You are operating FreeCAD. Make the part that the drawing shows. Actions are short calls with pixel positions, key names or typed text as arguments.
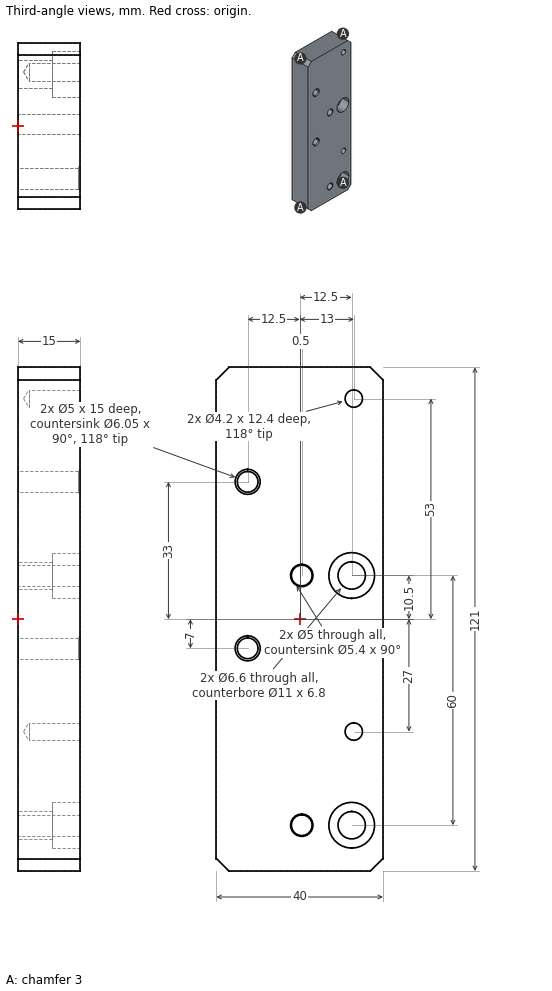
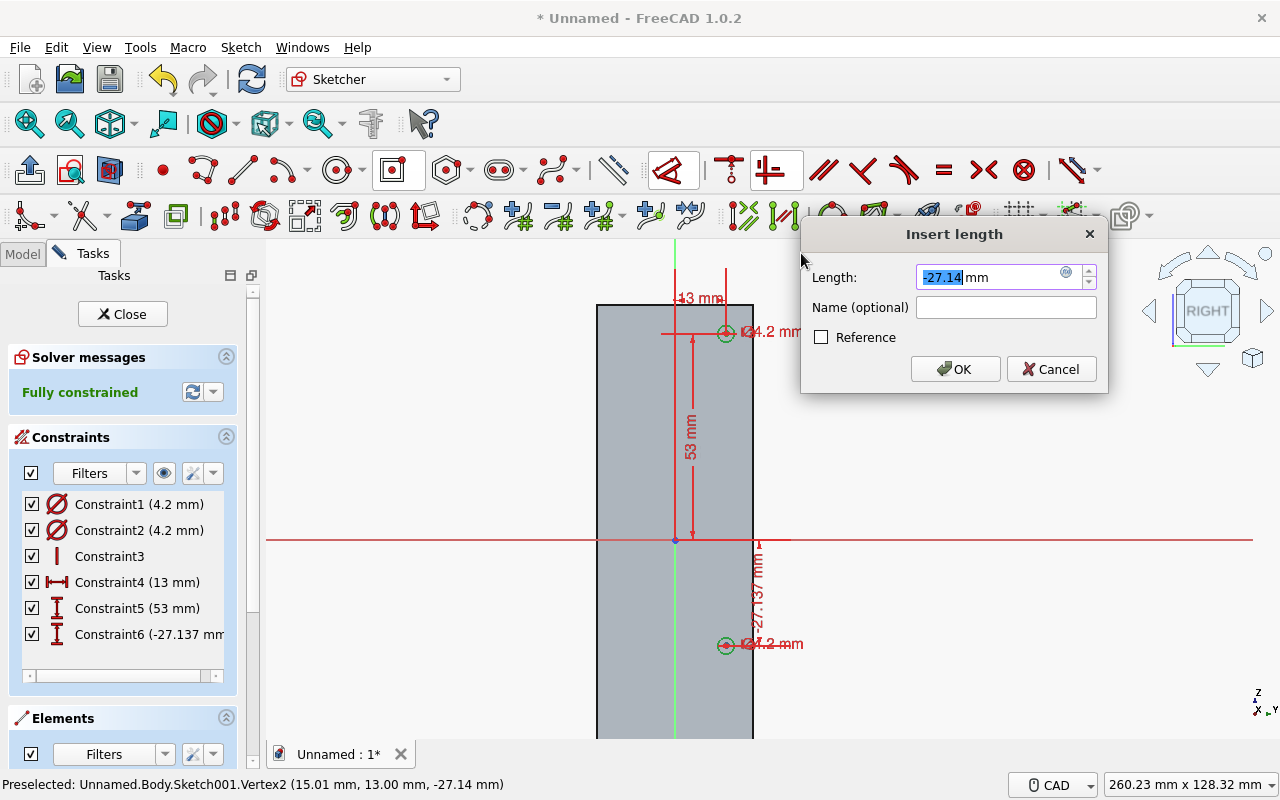
text(-27)
key(Return)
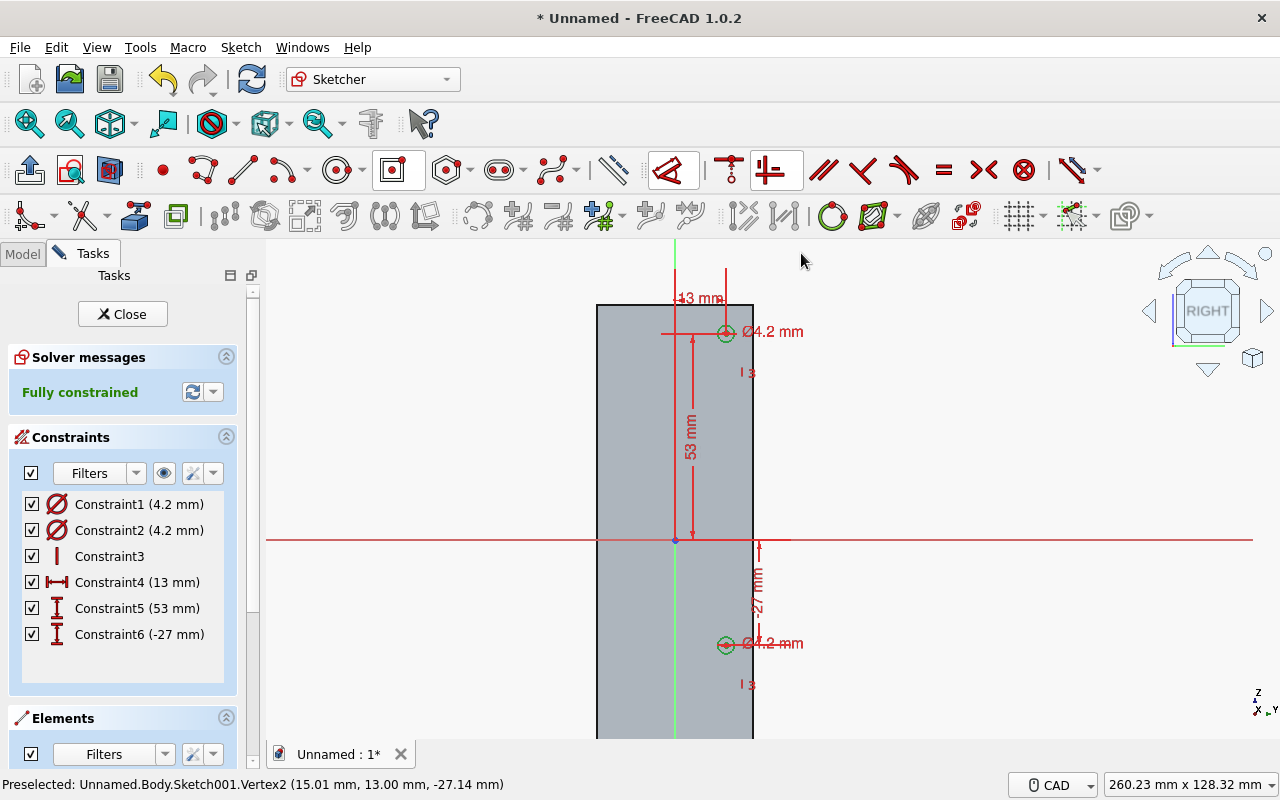
click(123, 314)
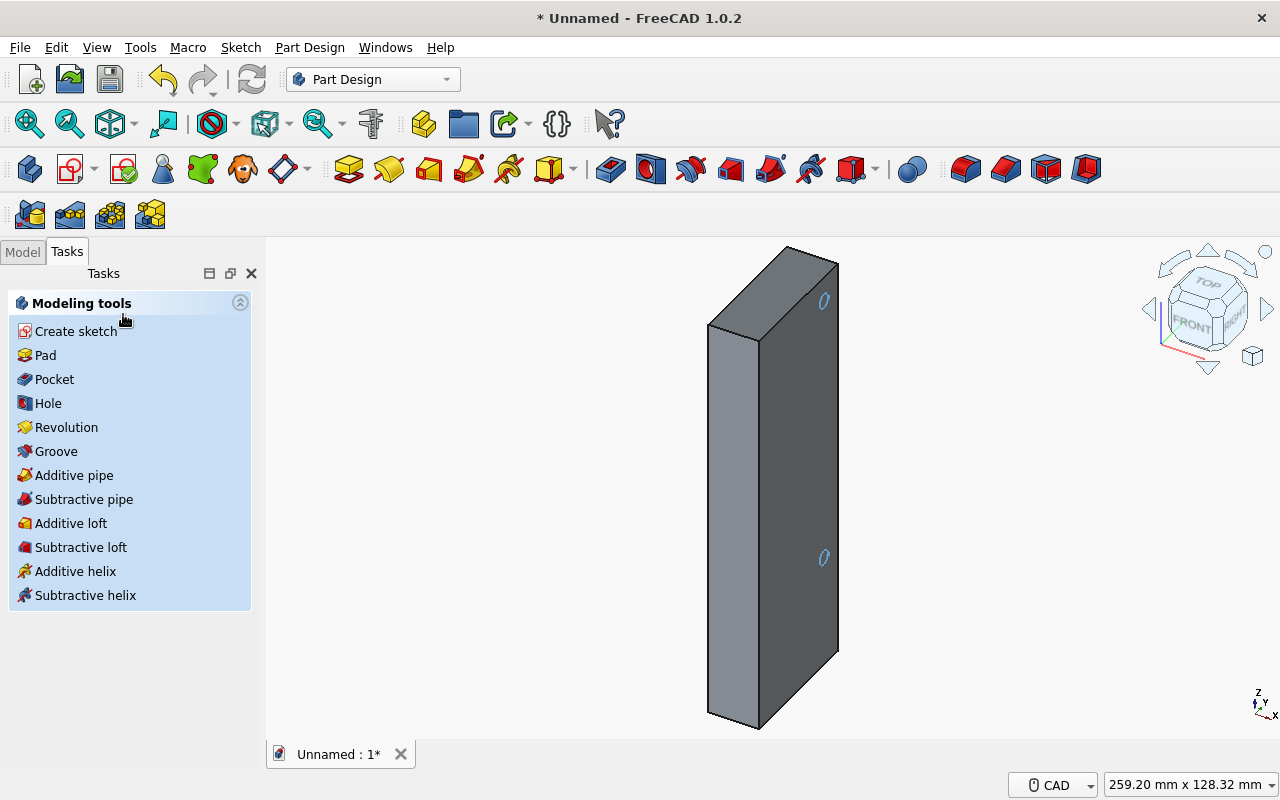
click(652, 170)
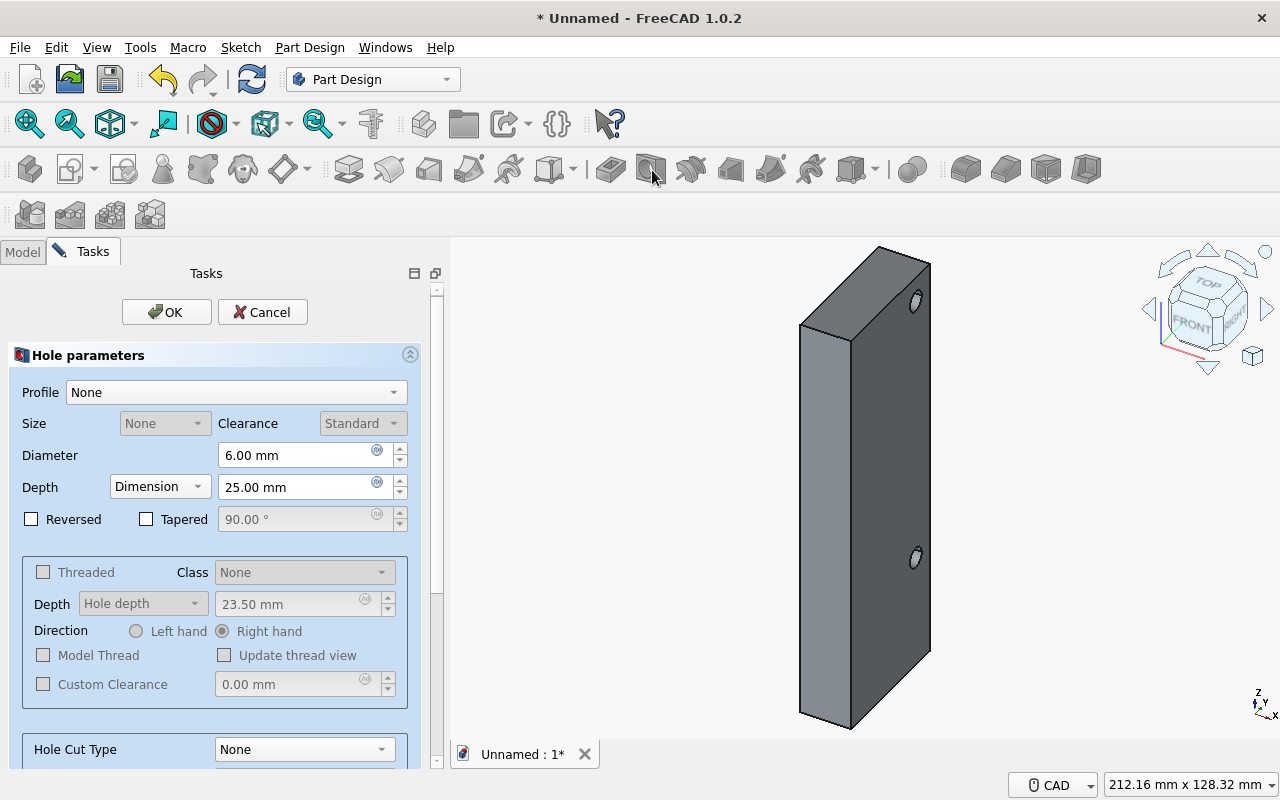
triple_click(305, 455)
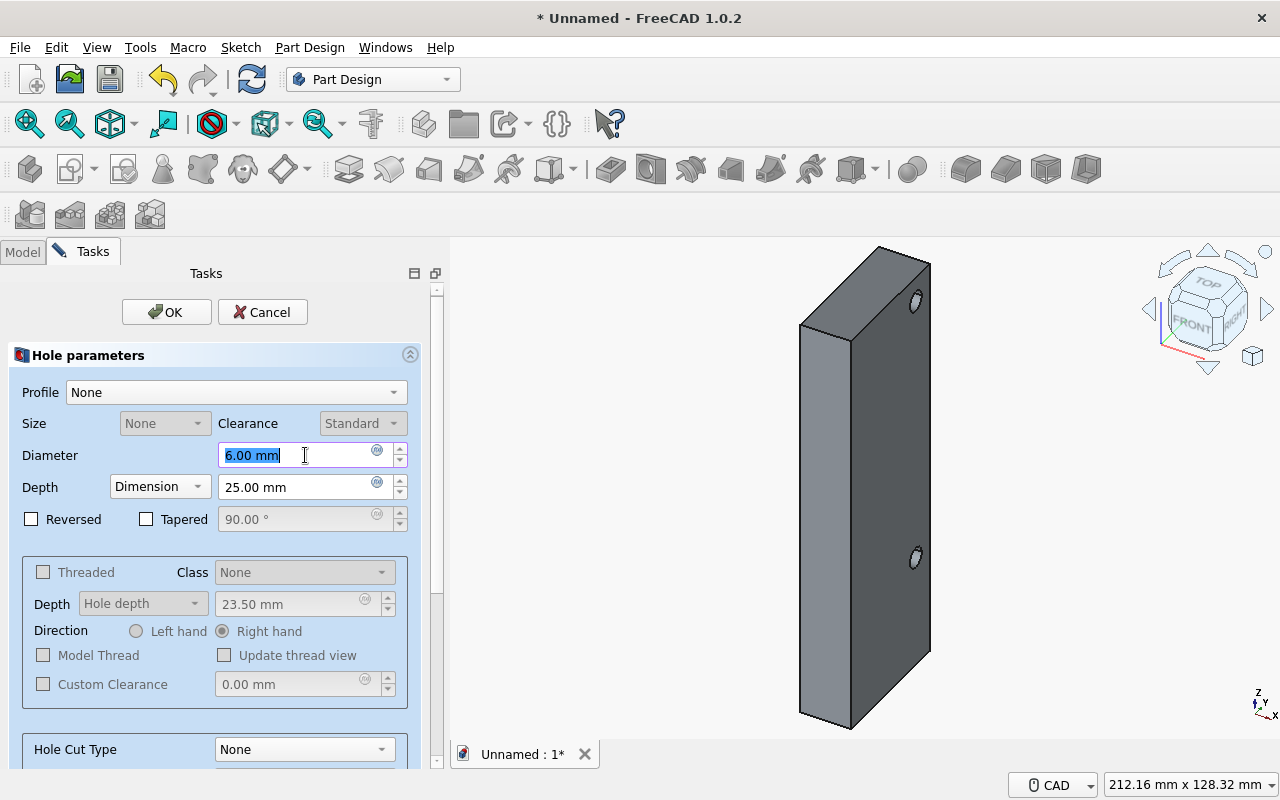
text(4.2)
key(Tab)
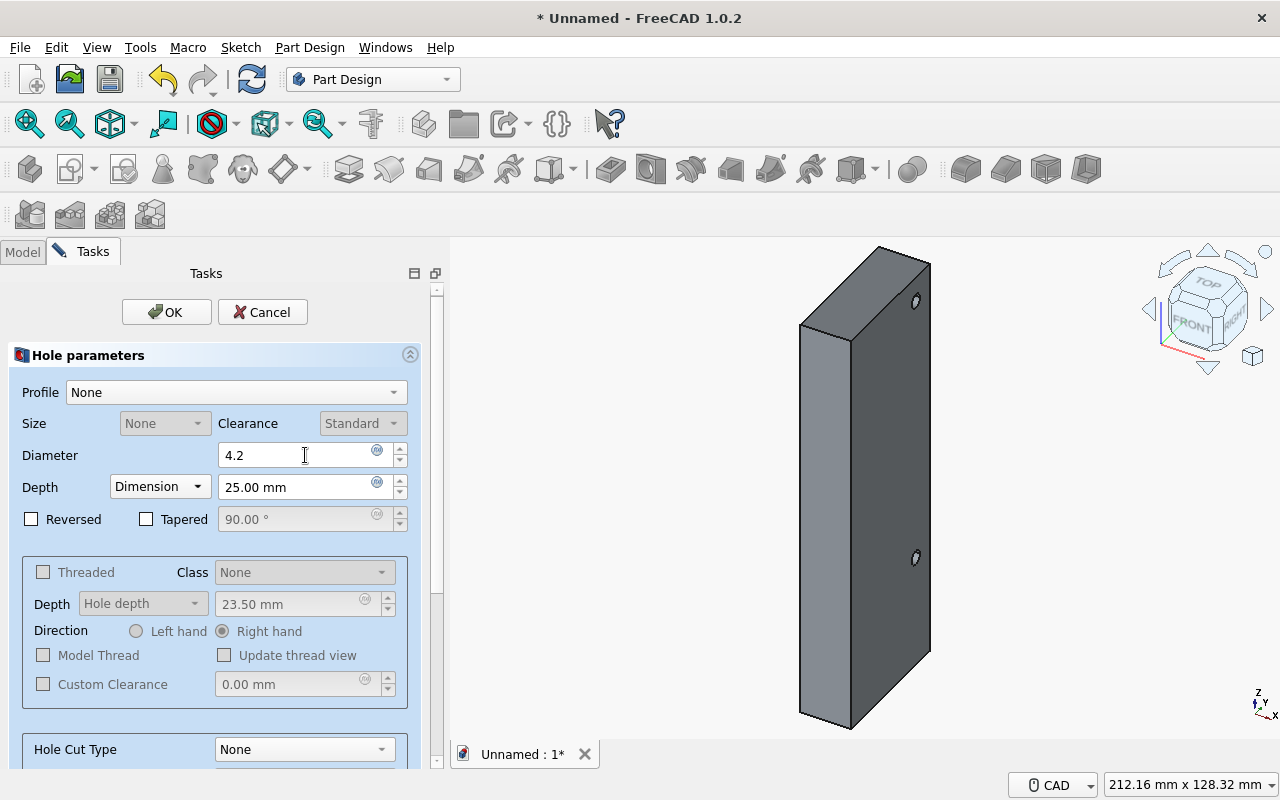
triple_click(305, 487)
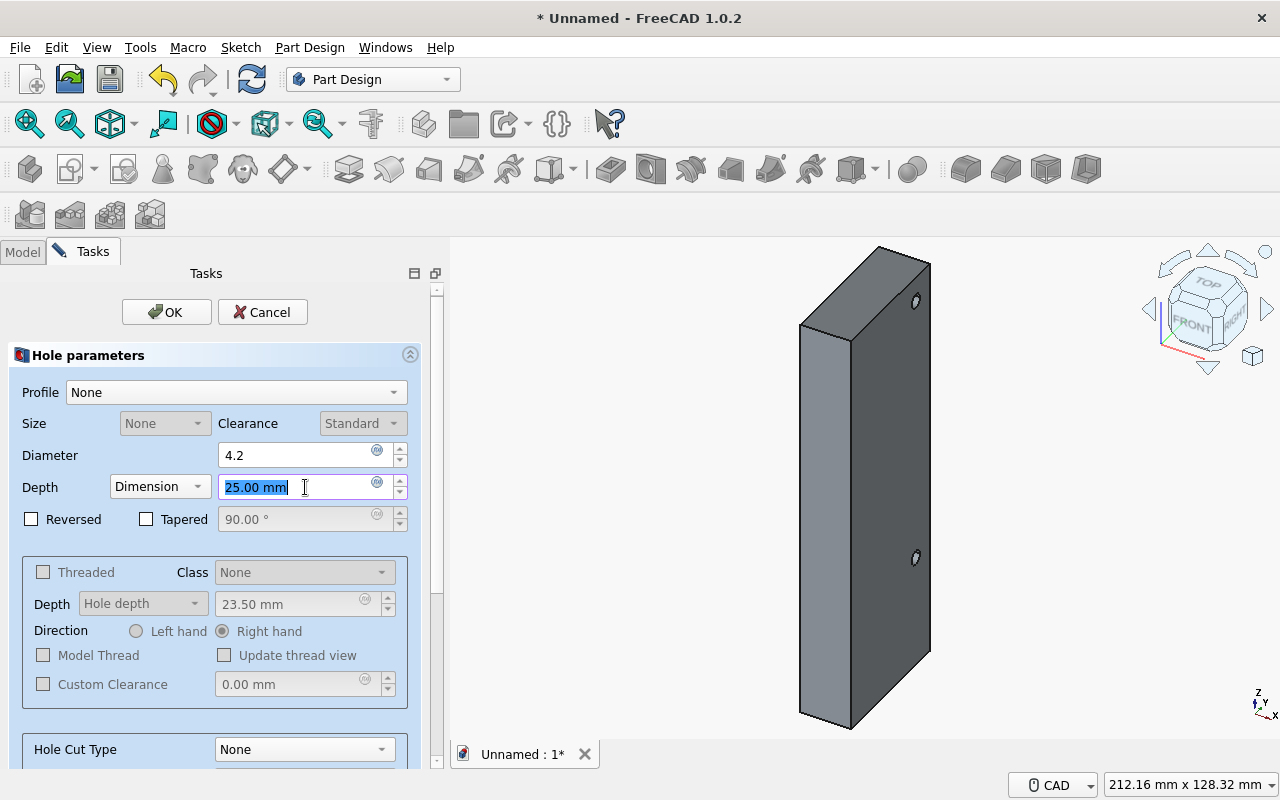
text(12.4)
key(Tab)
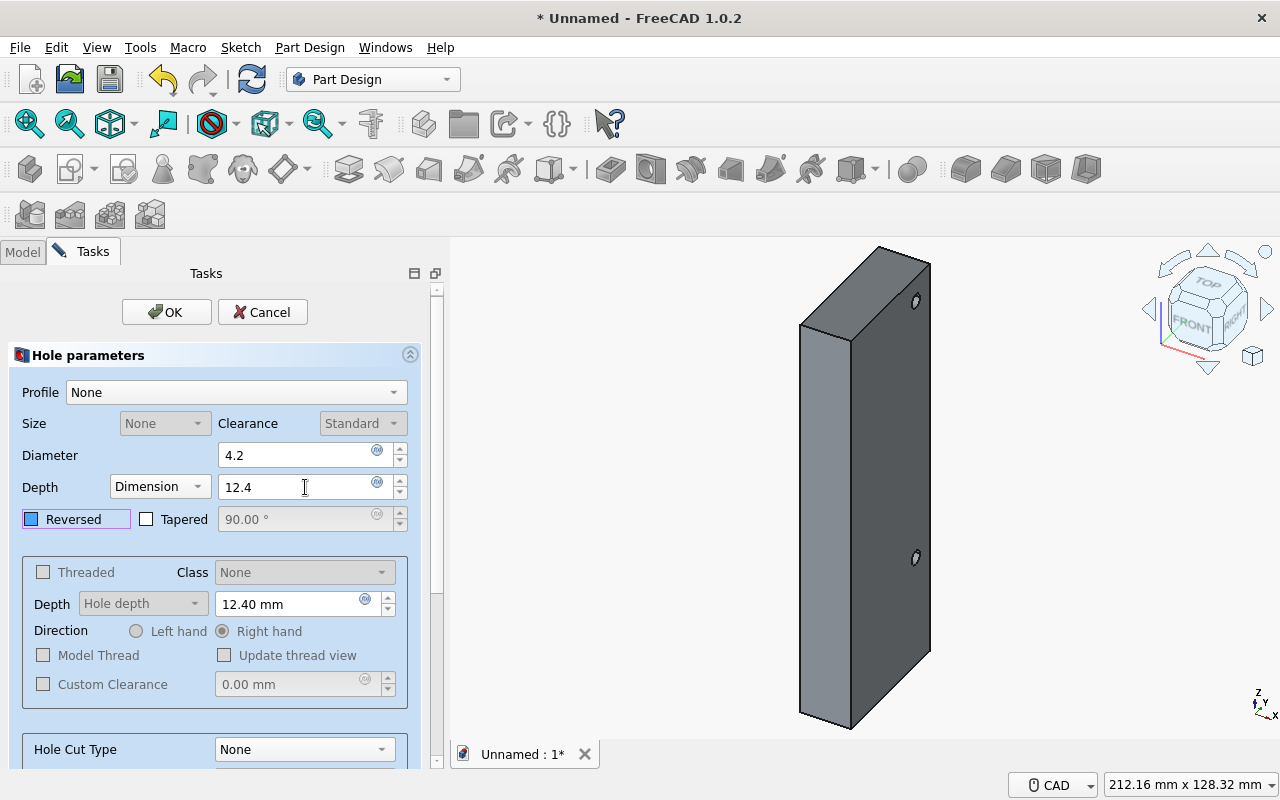
click(167, 312)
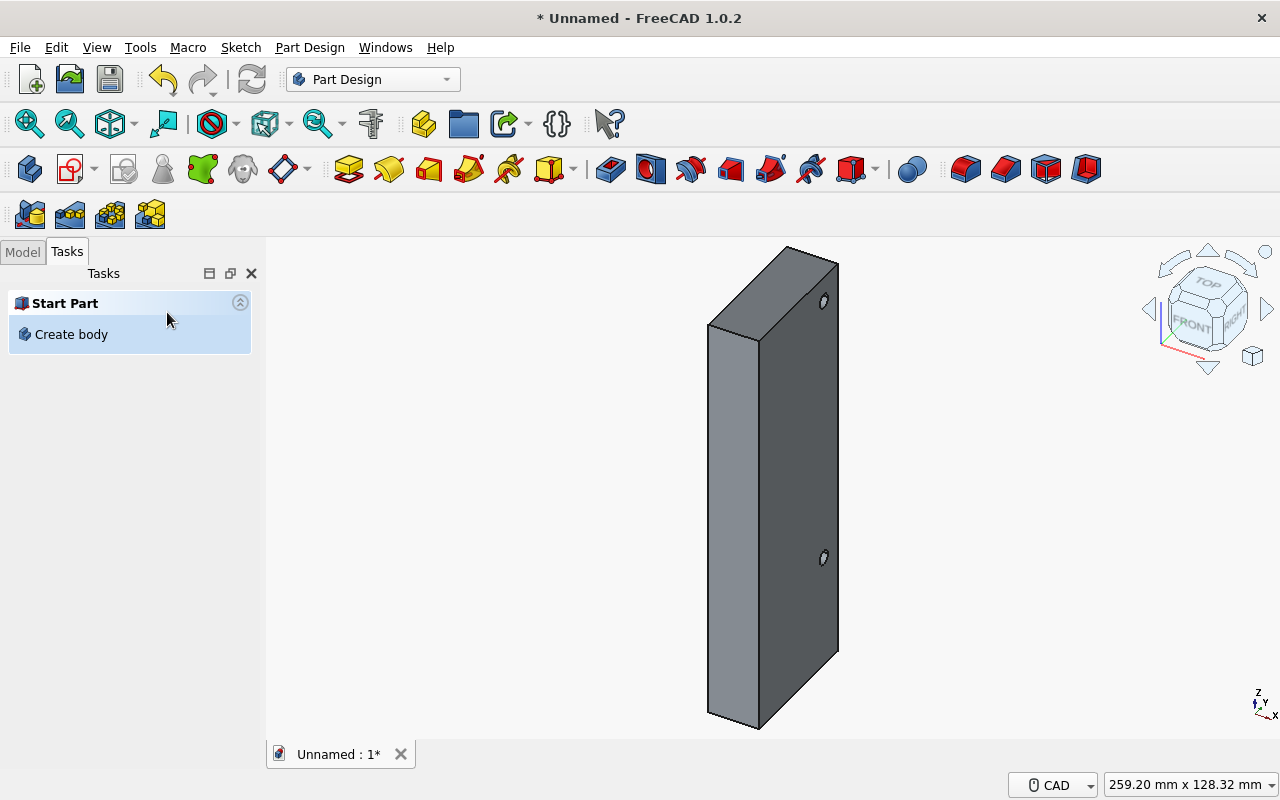
click(798, 495)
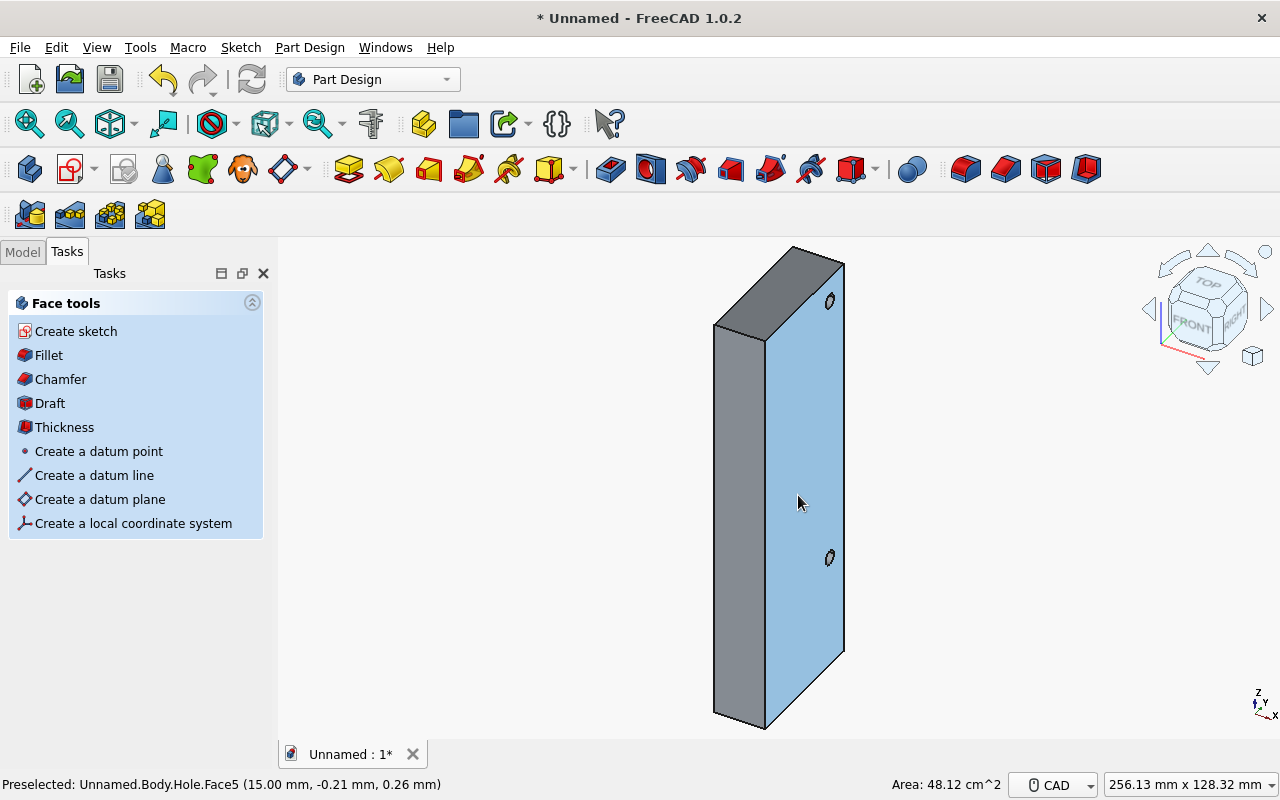
click(70, 170)